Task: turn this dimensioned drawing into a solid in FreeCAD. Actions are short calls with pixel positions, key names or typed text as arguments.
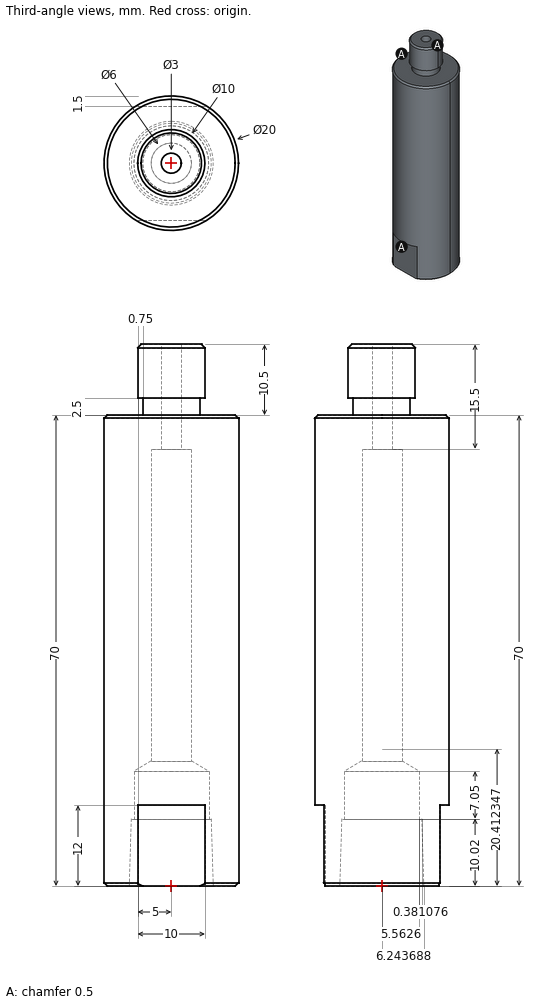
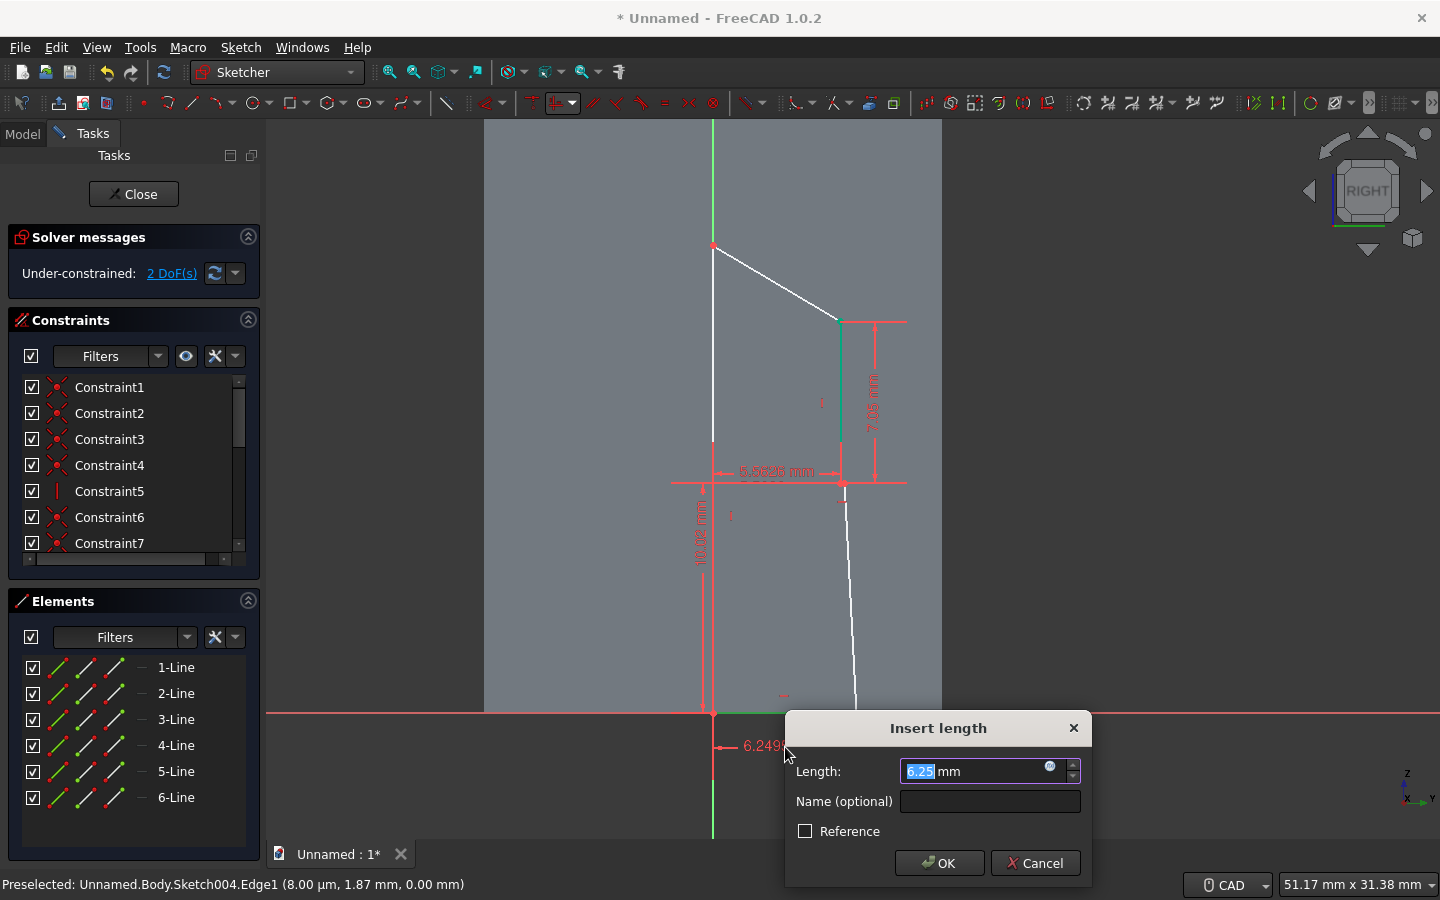
text(6.243688)
key(Return)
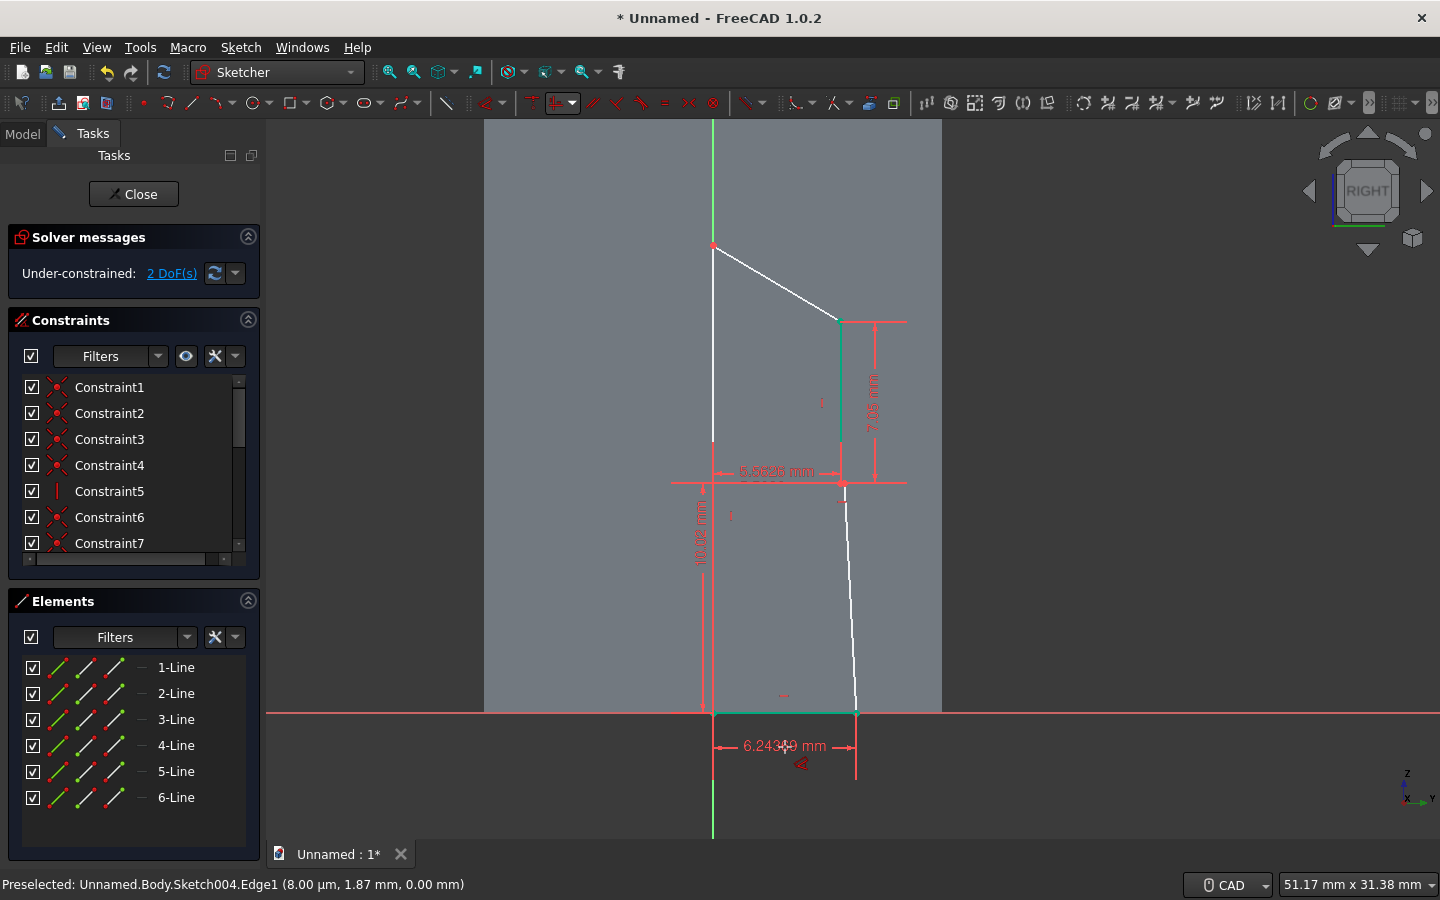
scroll(843, 483, up, 10)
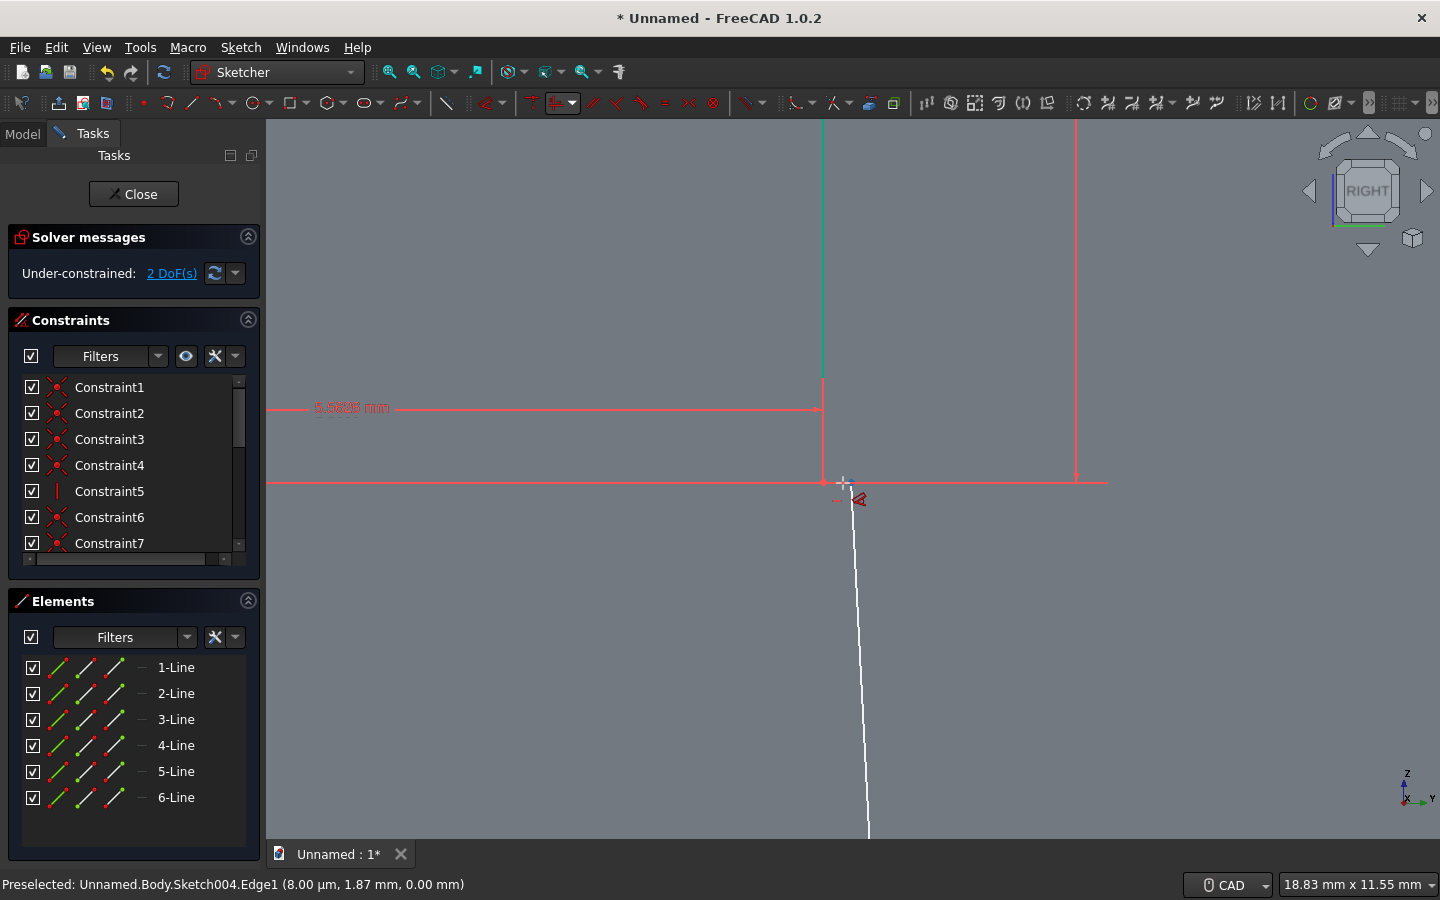
click(837, 483)
click(837, 517)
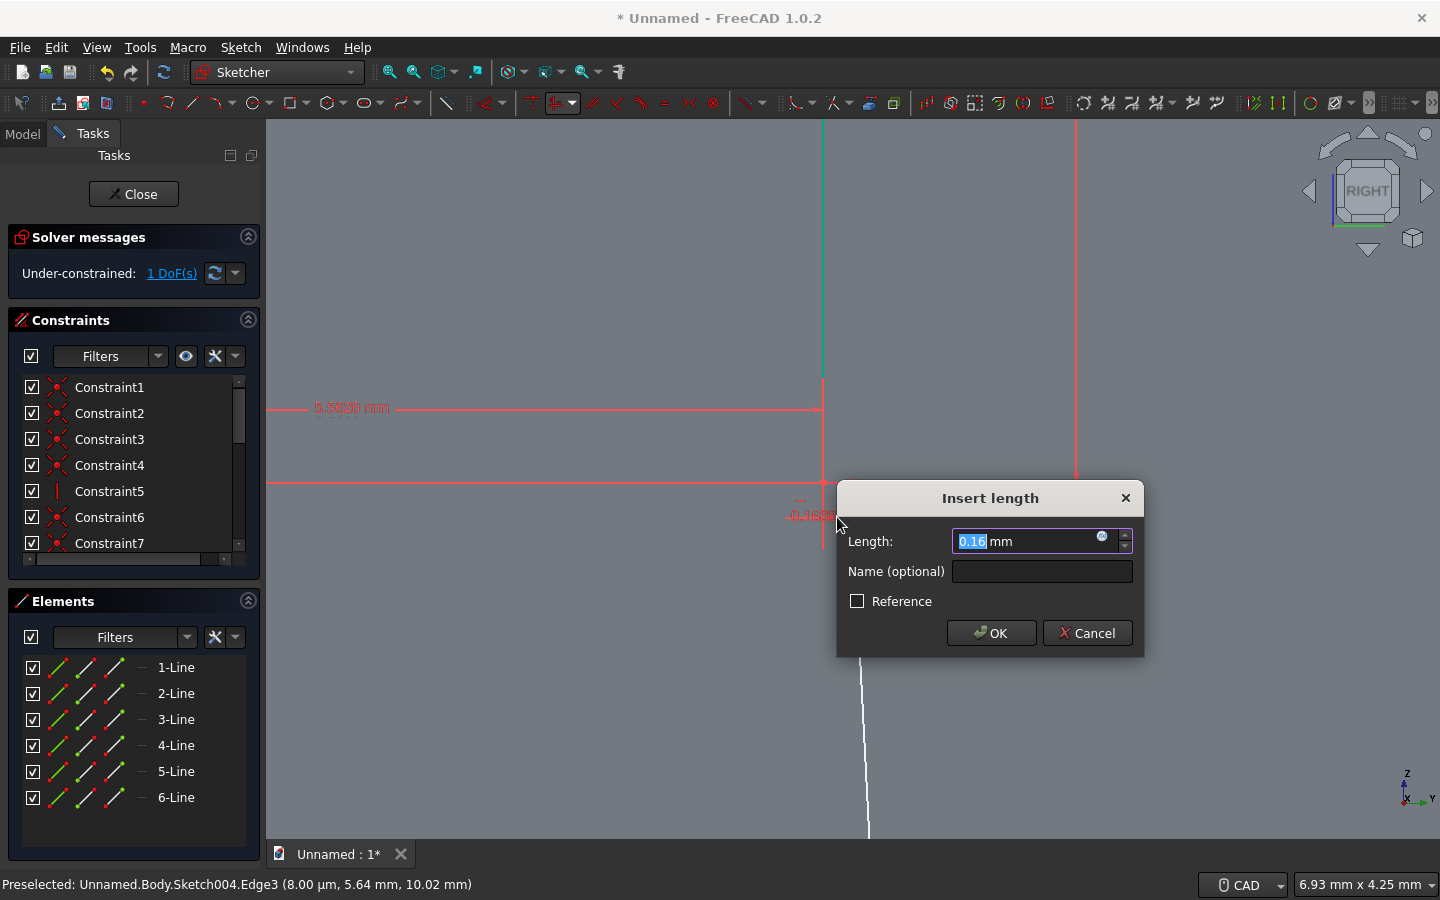
text(0.381076)
key(Return)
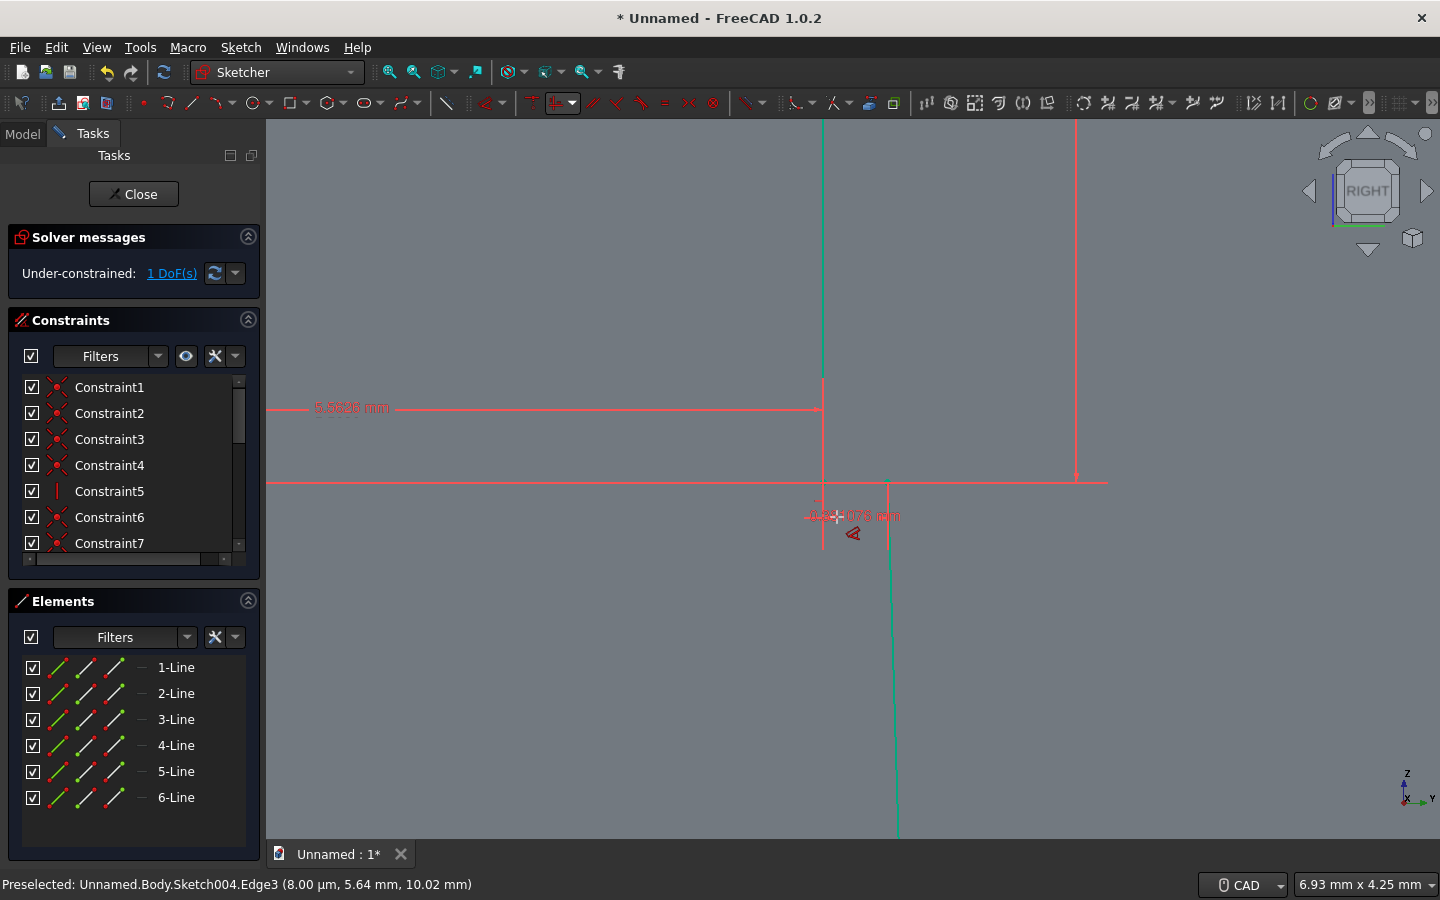
scroll(843, 483, down, 10)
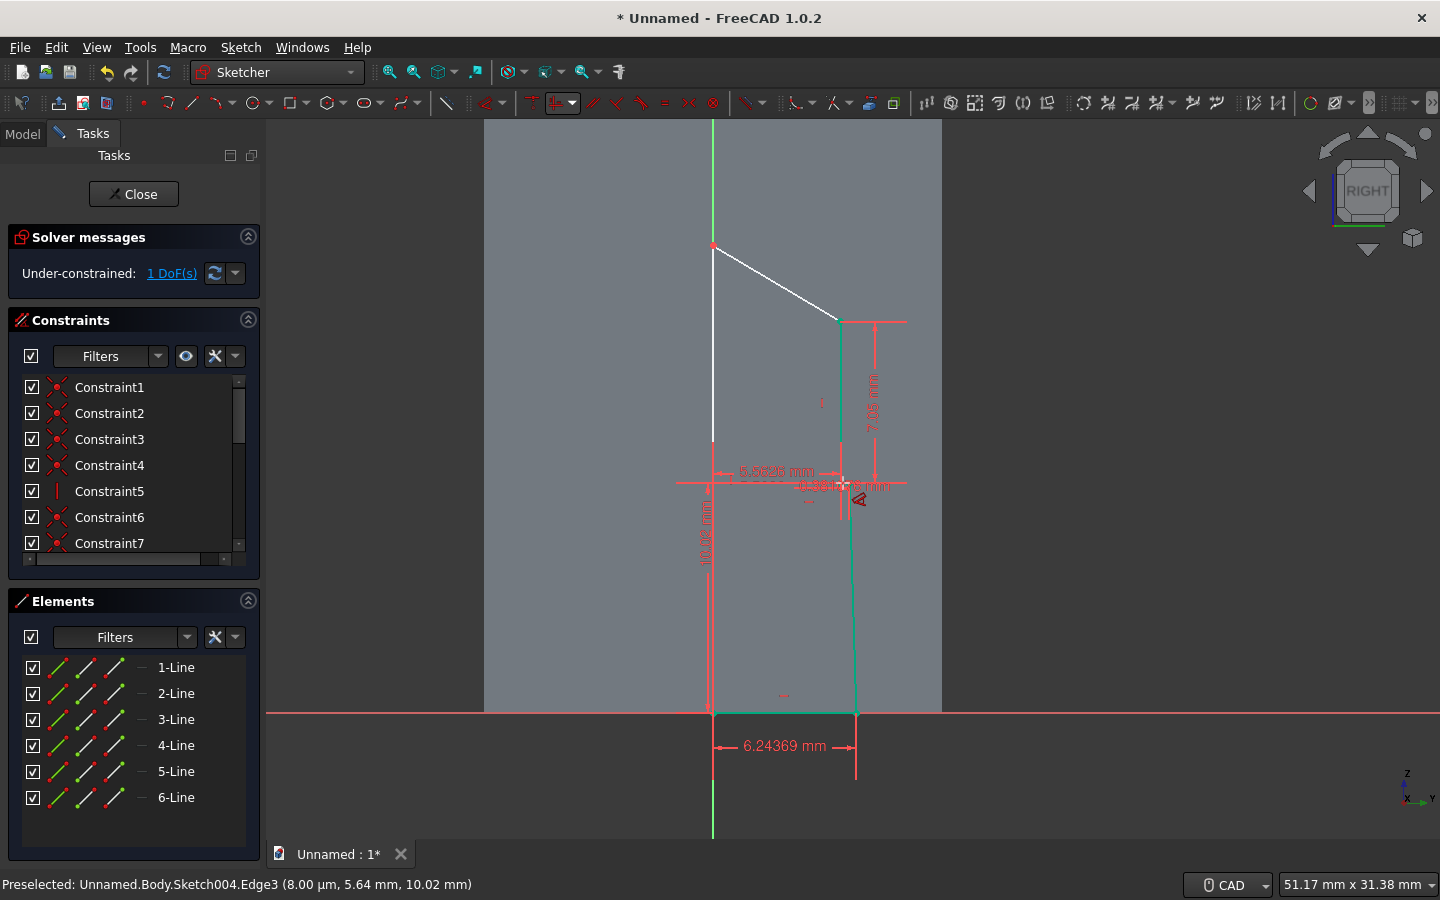
click(713, 386)
click(679, 480)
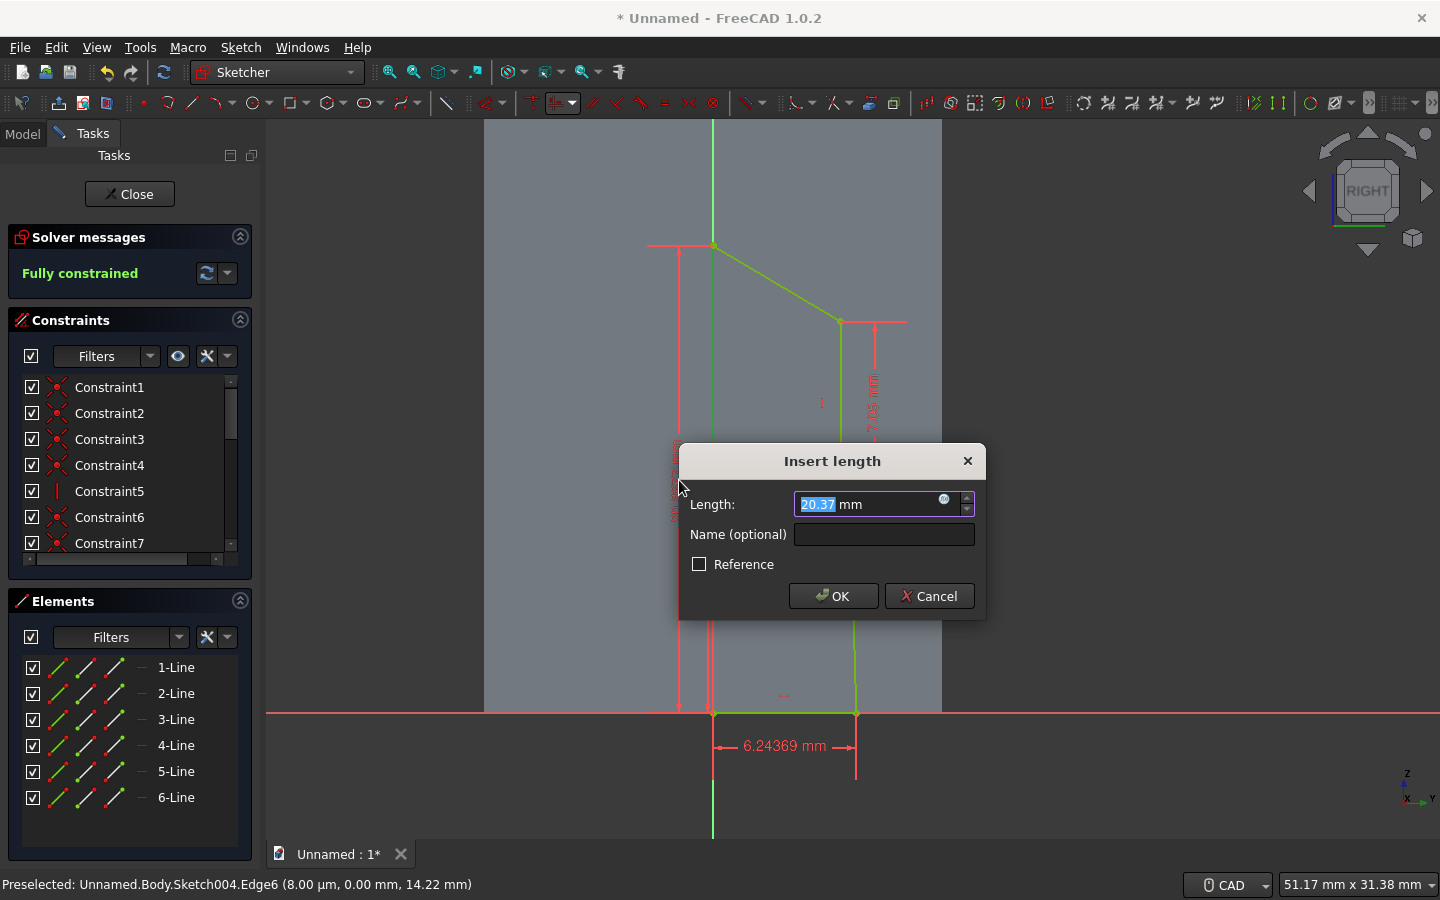
text(20.412347)
key(Return)
key(Escape)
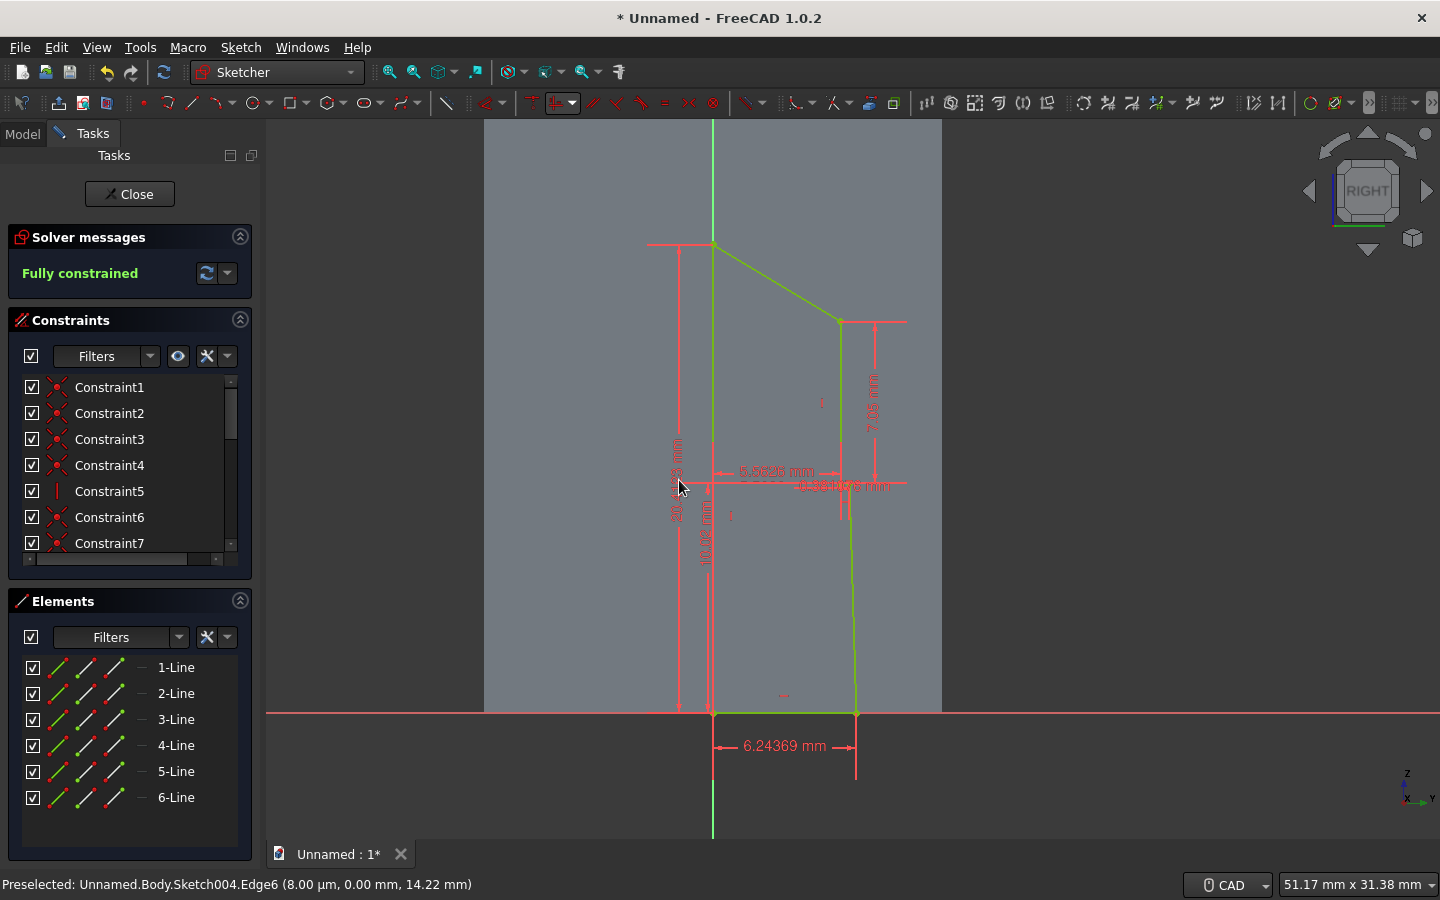
click(130, 194)